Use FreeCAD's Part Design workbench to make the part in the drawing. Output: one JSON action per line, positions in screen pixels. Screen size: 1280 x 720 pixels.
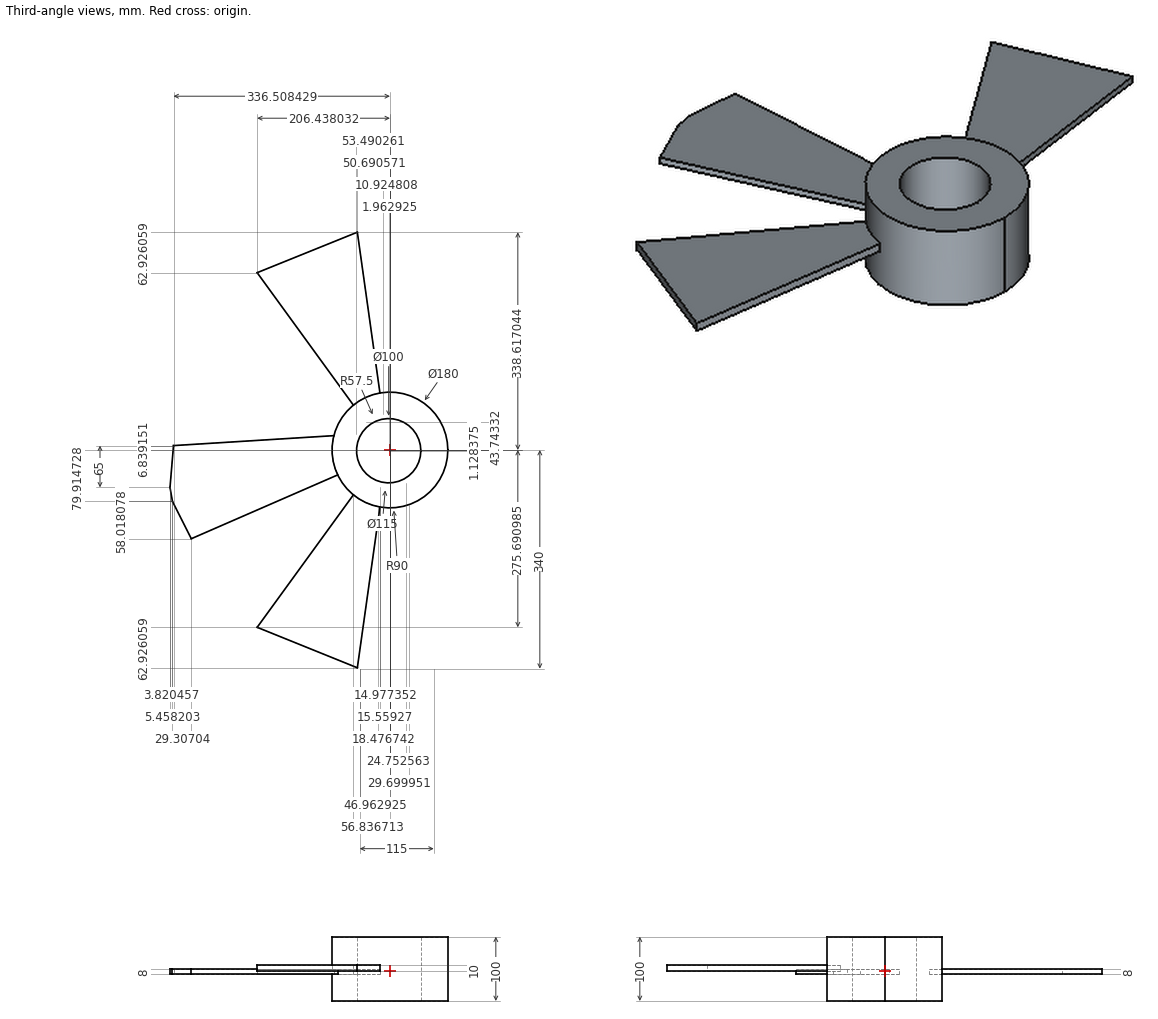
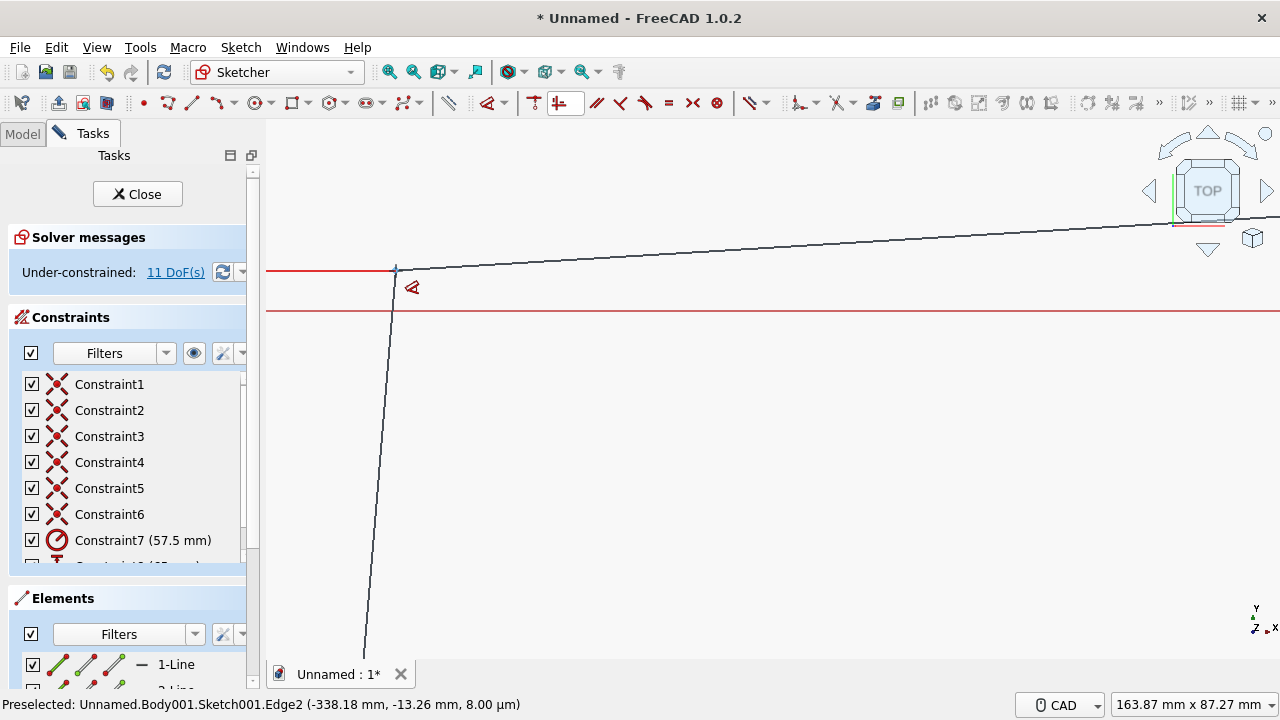
{"action": "left_click", "coordinate": [396, 271]}
{"action": "left_click", "coordinate": [362, 291]}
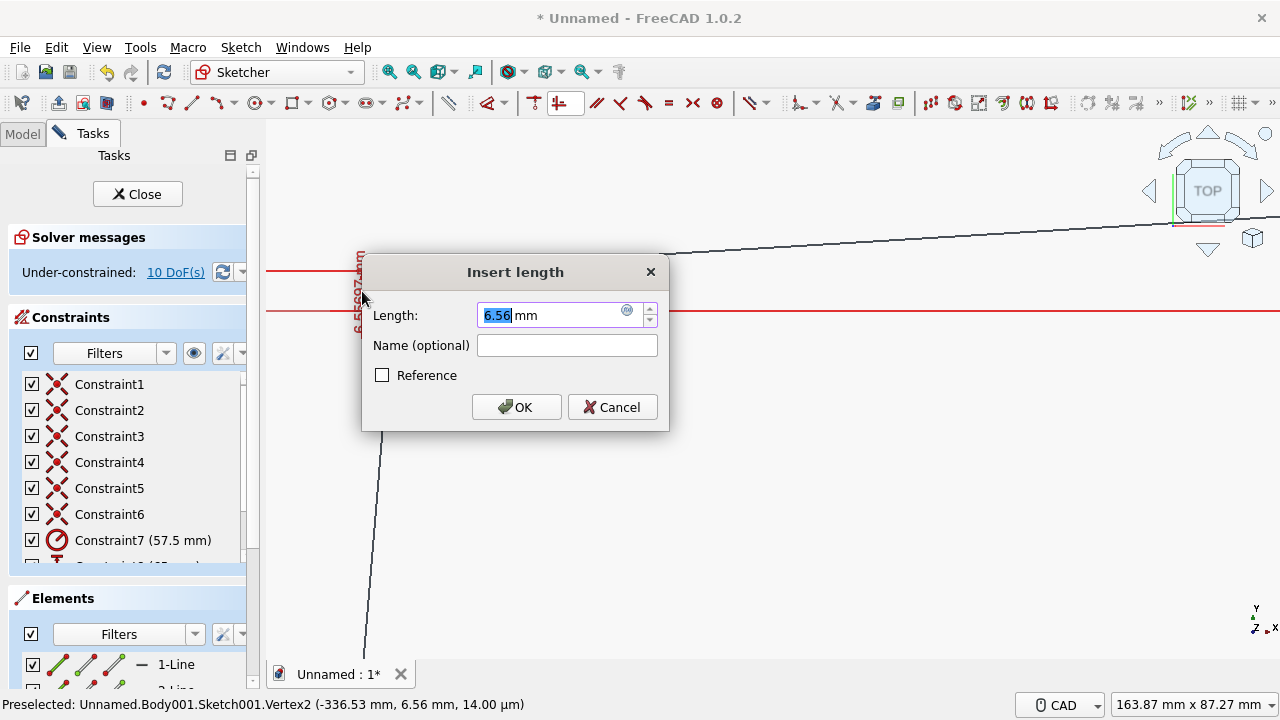
{"action": "type", "text": "6.839151"}
{"action": "key", "text": "Return"}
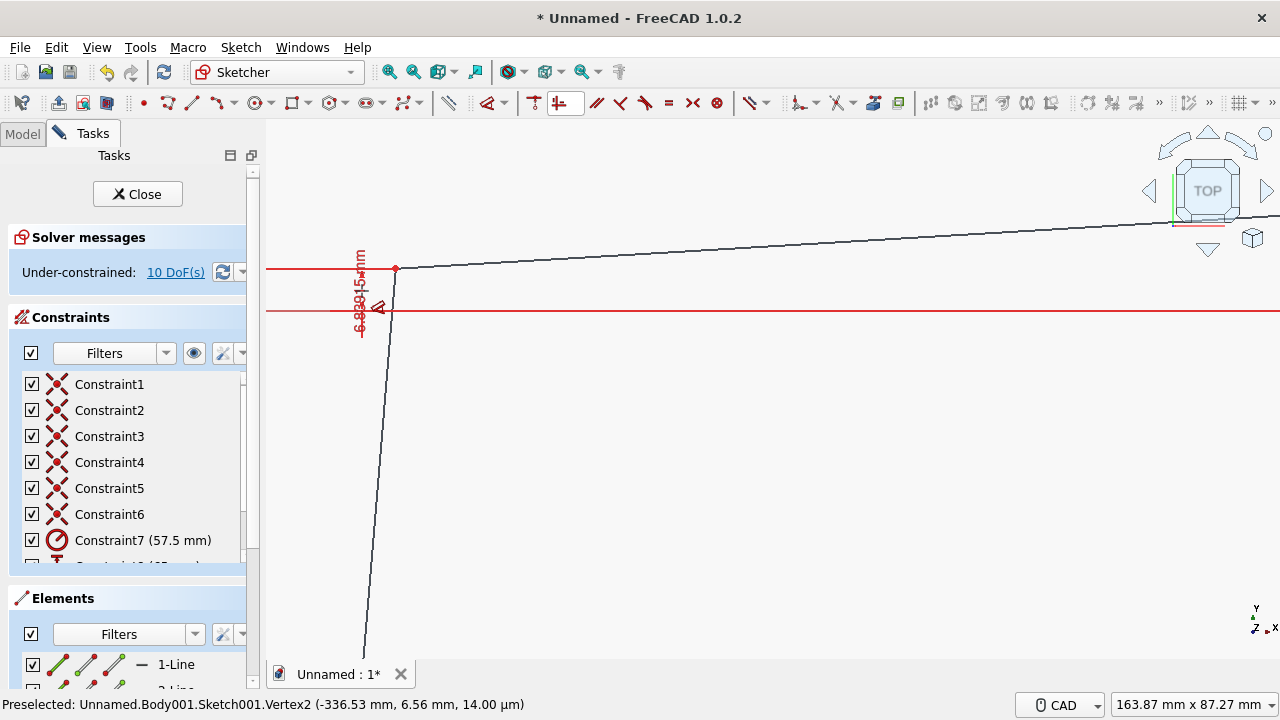
{"action": "left_click", "coordinate": [386, 389]}
{"action": "left_click", "coordinate": [379, 235]}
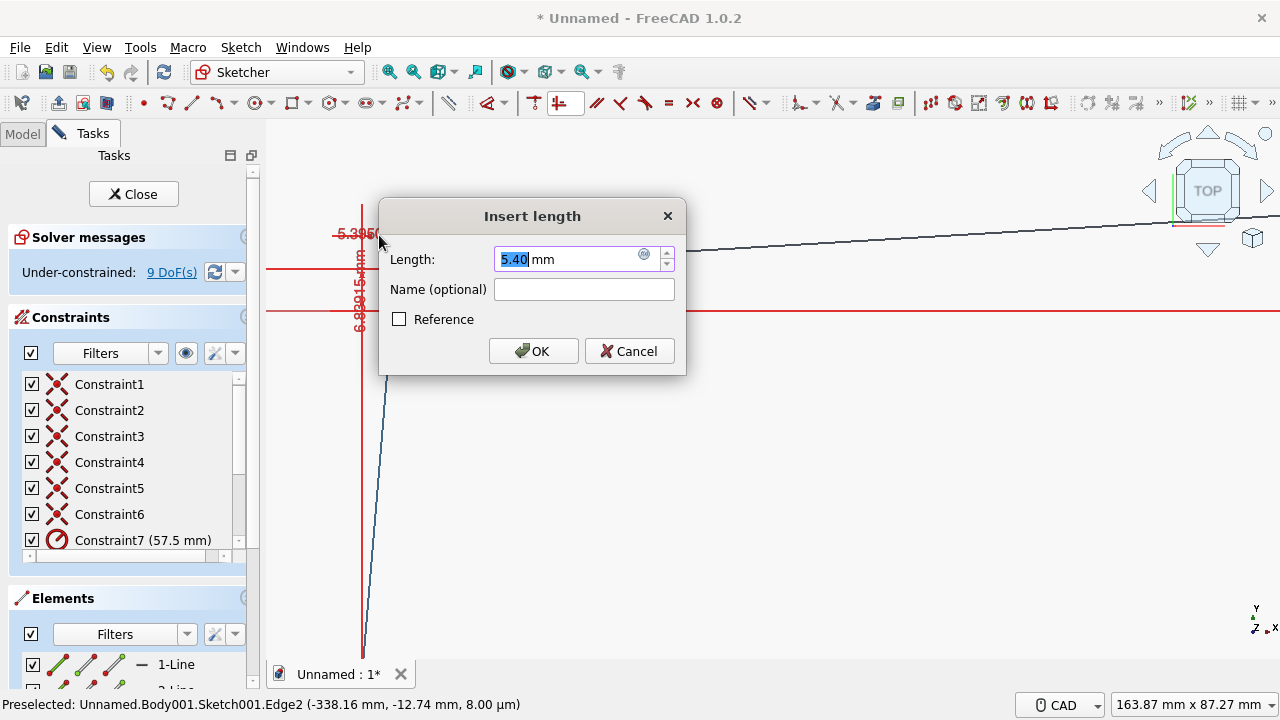
{"action": "type", "text": "5.458203"}
{"action": "key", "text": "Return"}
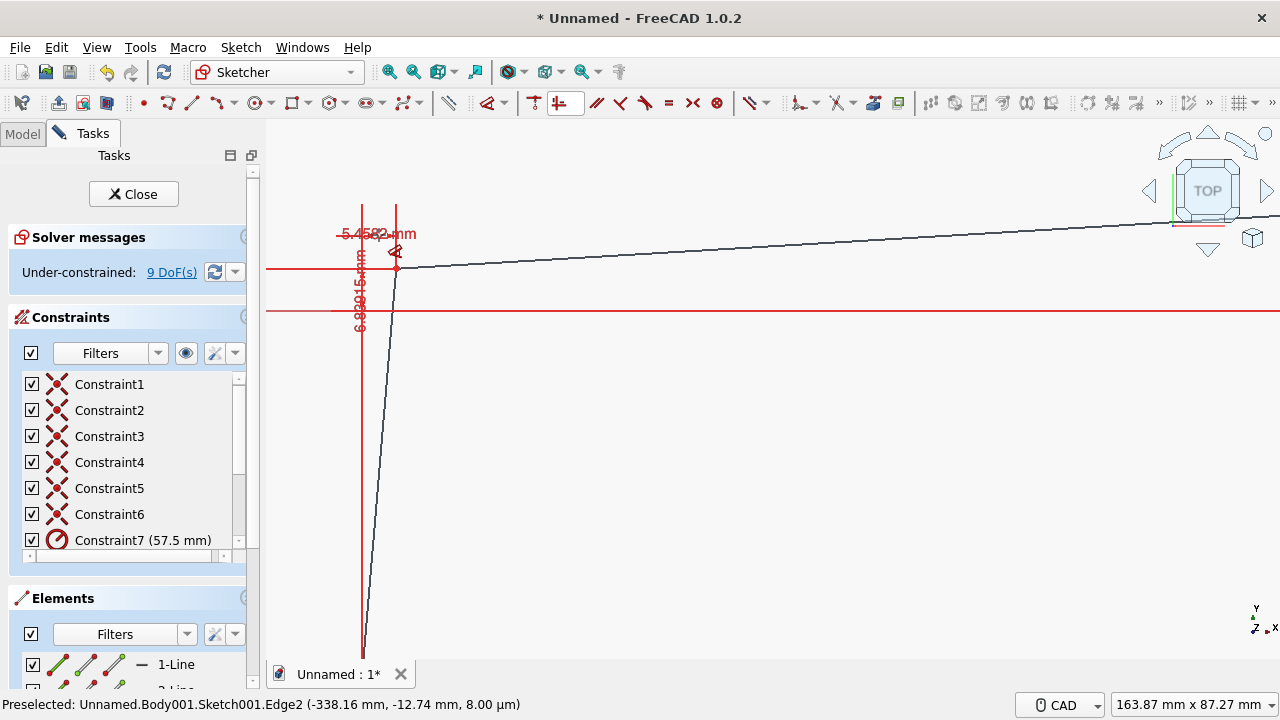
{"action": "scroll", "coordinate": [396, 271], "scroll_direction": "down", "scroll_amount": 6}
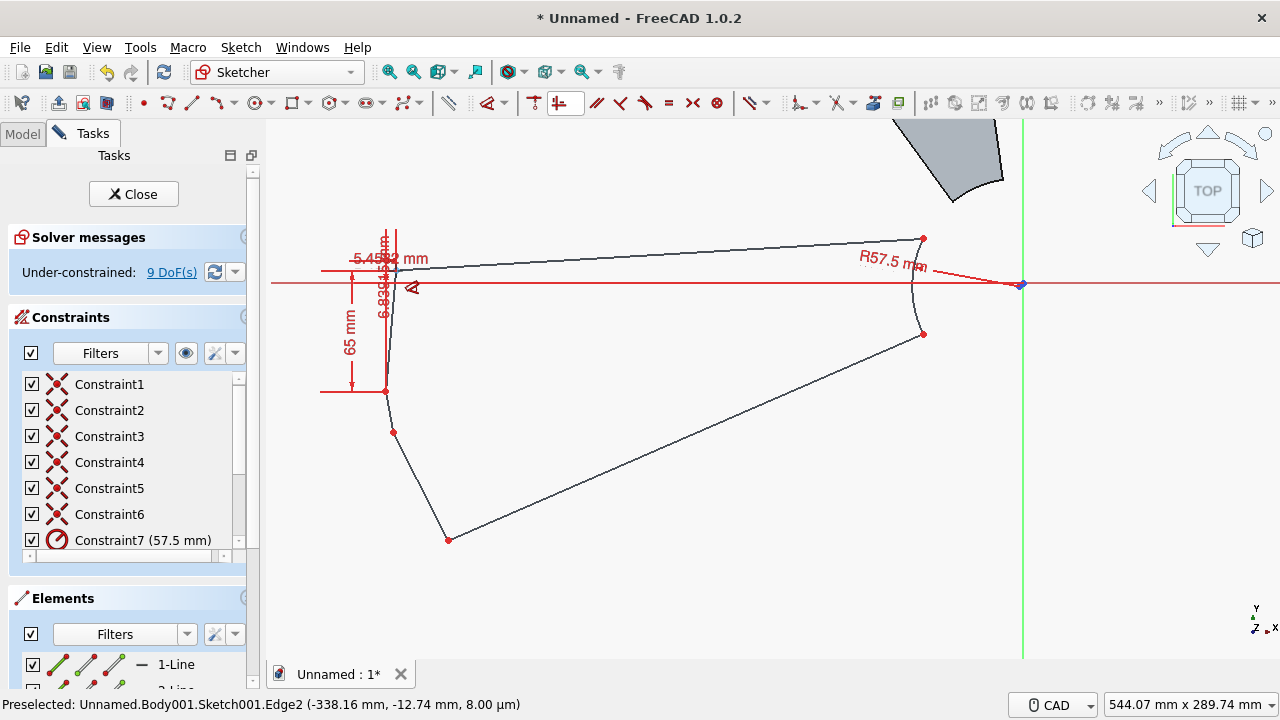
{"action": "scroll", "coordinate": [388, 404], "scroll_direction": "up", "scroll_amount": 9}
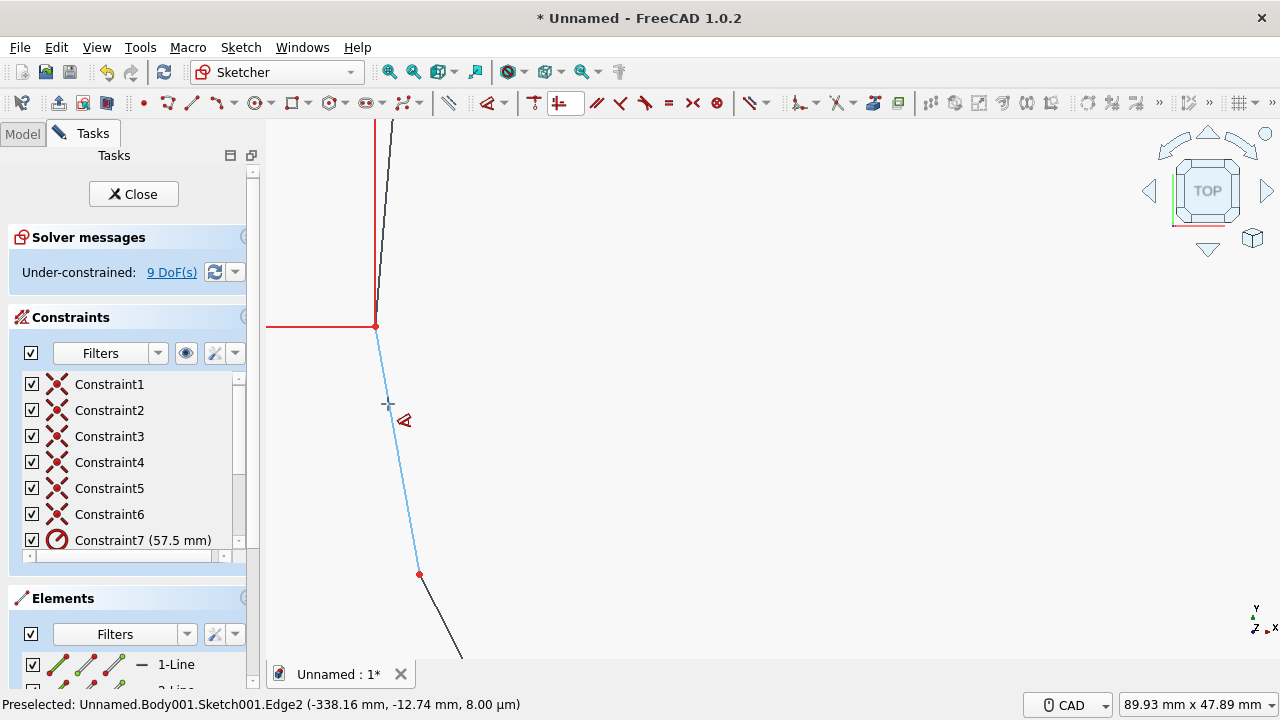
{"action": "left_click", "coordinate": [389, 401]}
{"action": "left_click", "coordinate": [398, 608]}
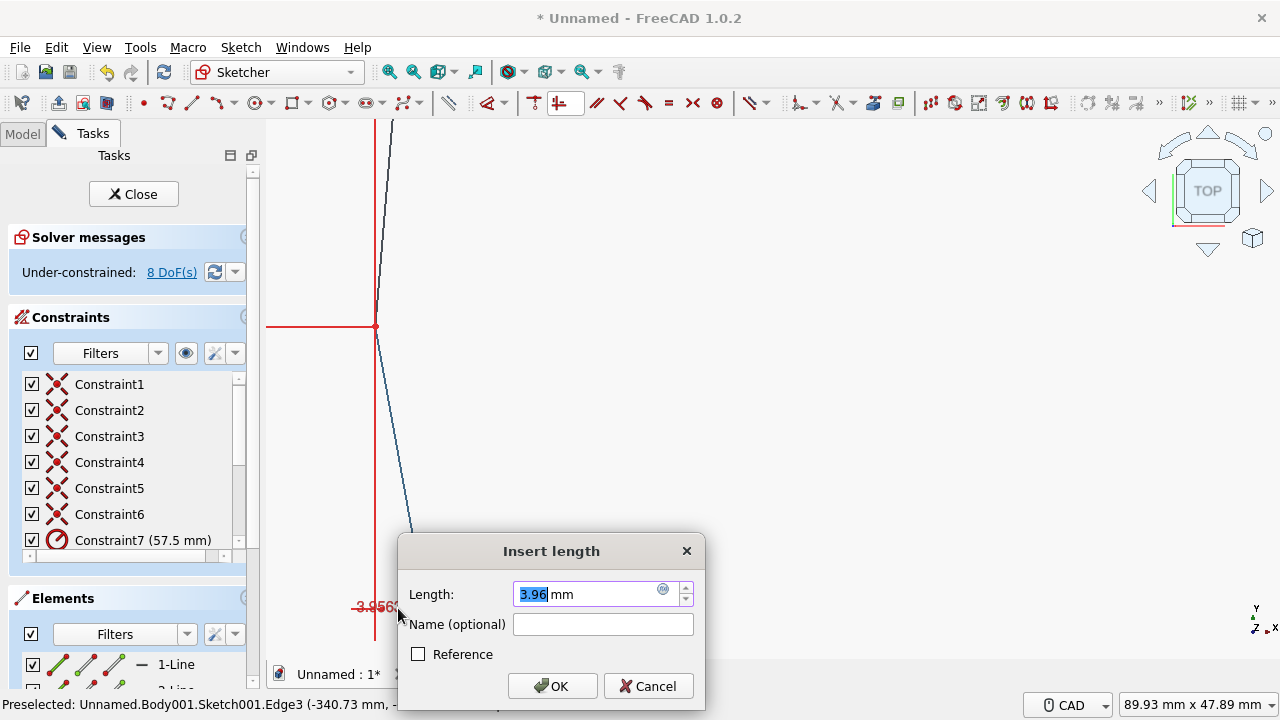
{"action": "type", "text": "3.820457"}
{"action": "key", "text": "Return"}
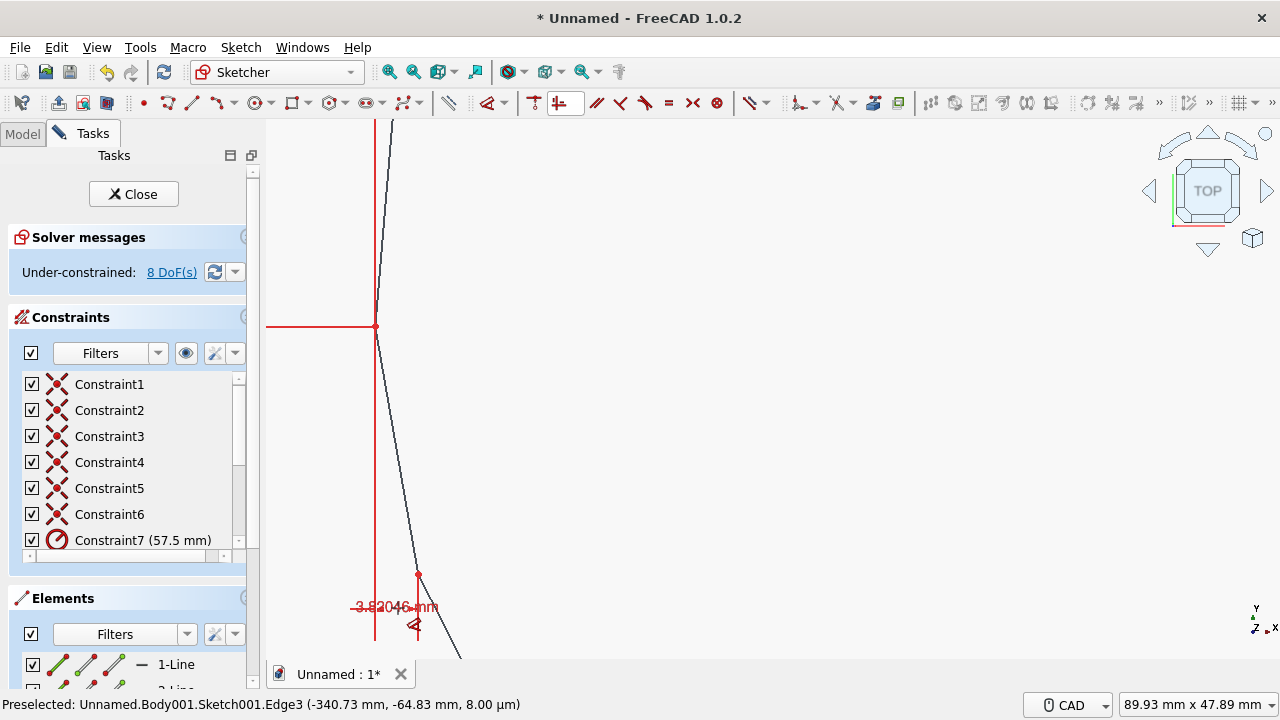
{"action": "scroll", "coordinate": [388, 404], "scroll_direction": "down", "scroll_amount": 9}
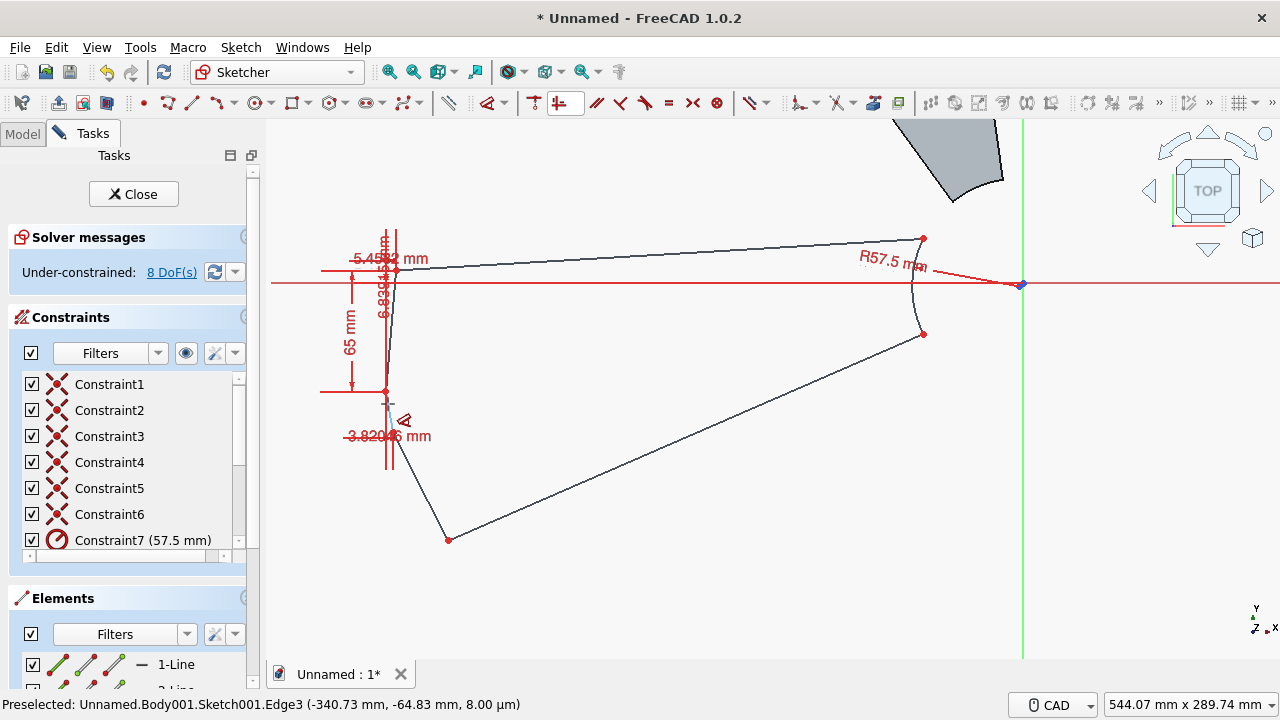
{"action": "left_click", "coordinate": [410, 465]}
{"action": "left_click", "coordinate": [421, 575]}